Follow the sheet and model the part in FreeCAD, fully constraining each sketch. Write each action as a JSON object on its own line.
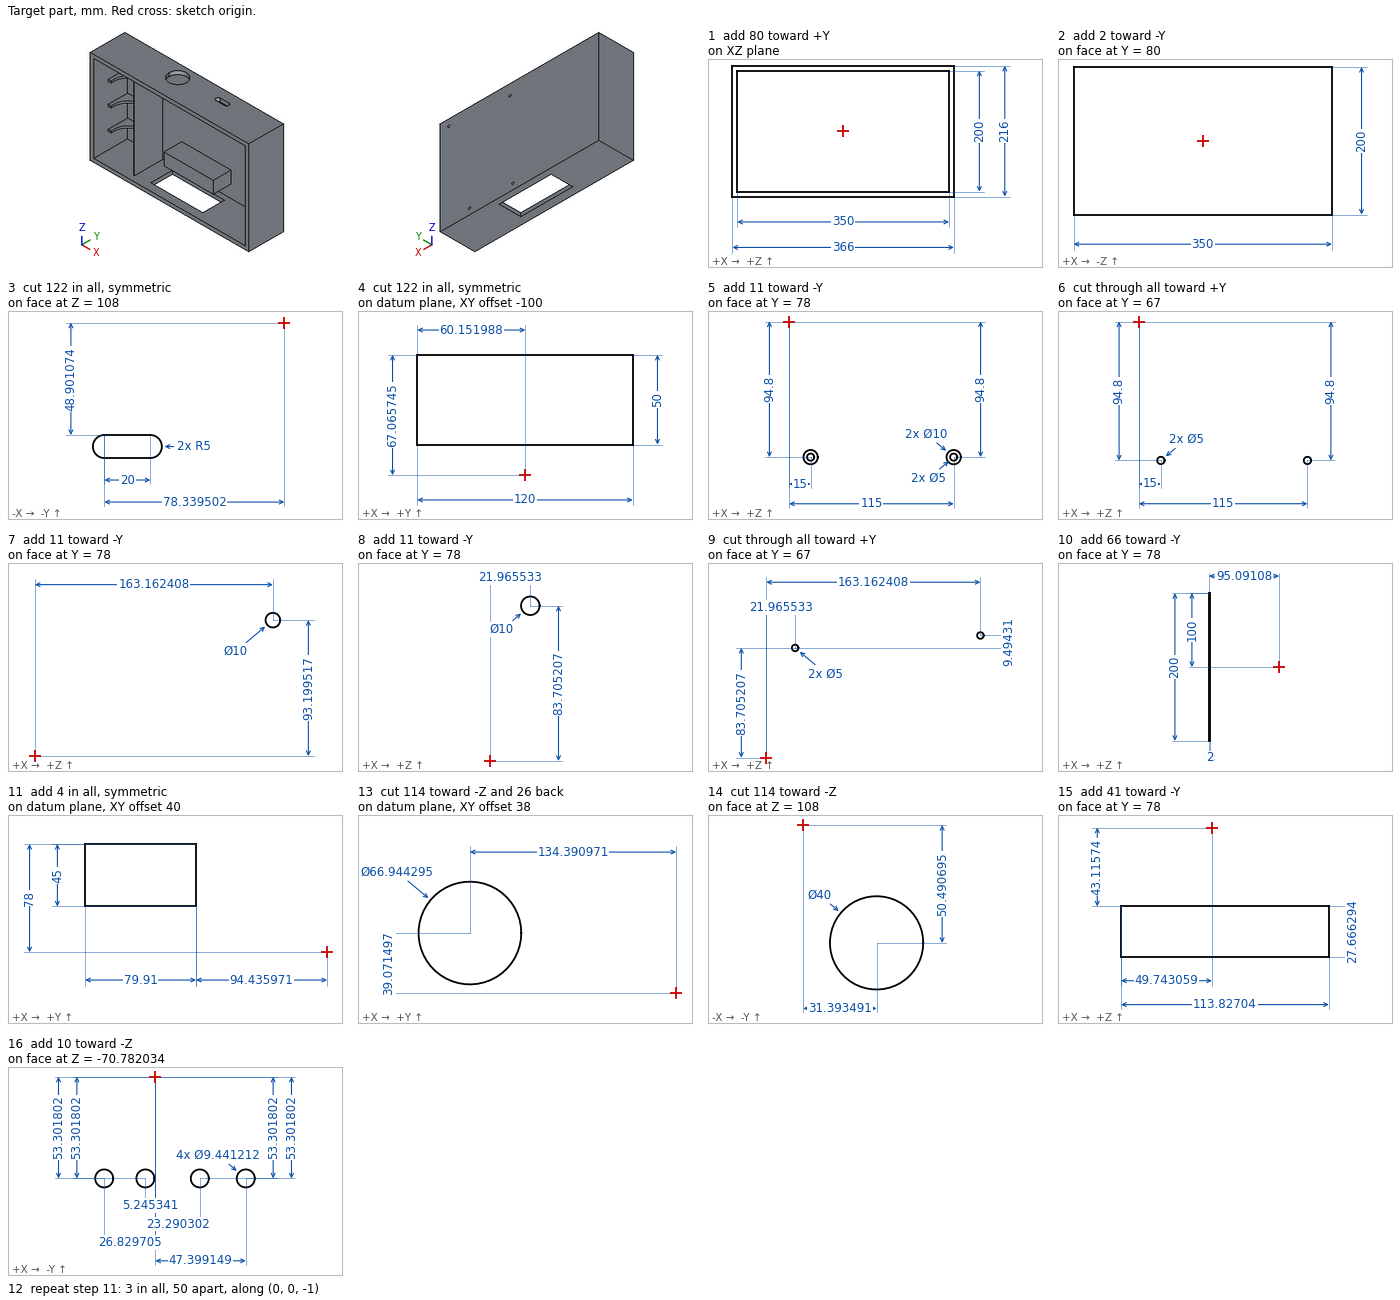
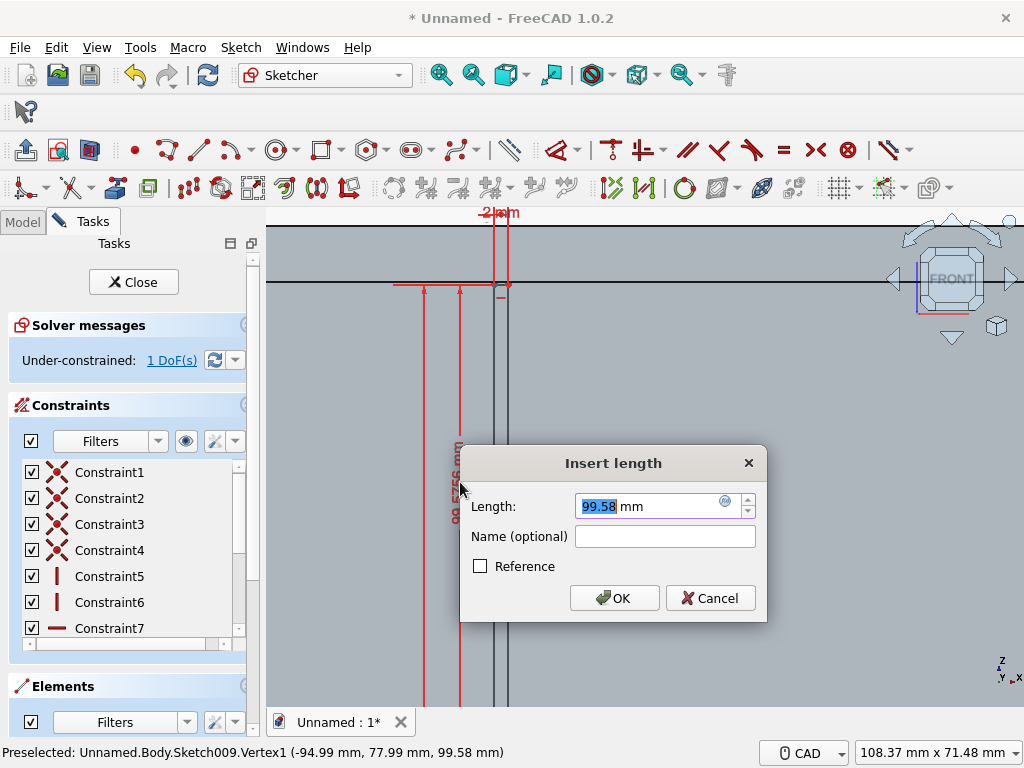
{"action": "type", "text": "100"}
{"action": "key", "text": "Return"}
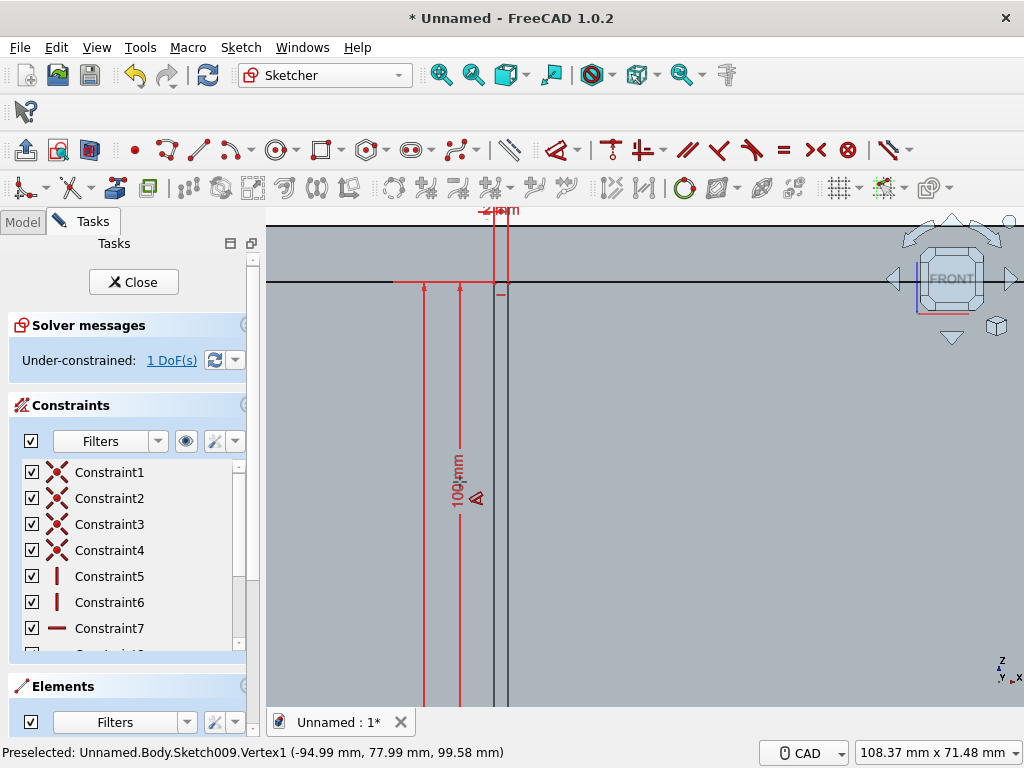
{"action": "left_click", "coordinate": [494, 282]}
{"action": "left_click", "coordinate": [677, 248]}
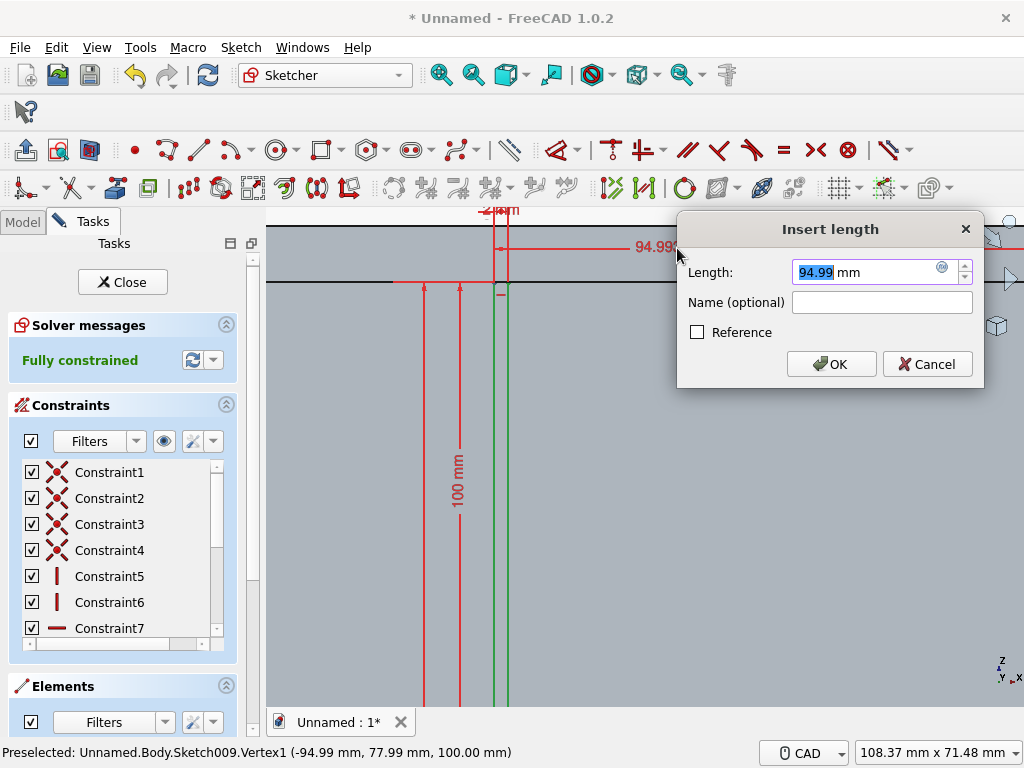
{"action": "type", "text": "95.09108"}
{"action": "key", "text": "Return"}
{"action": "key", "text": "Escape"}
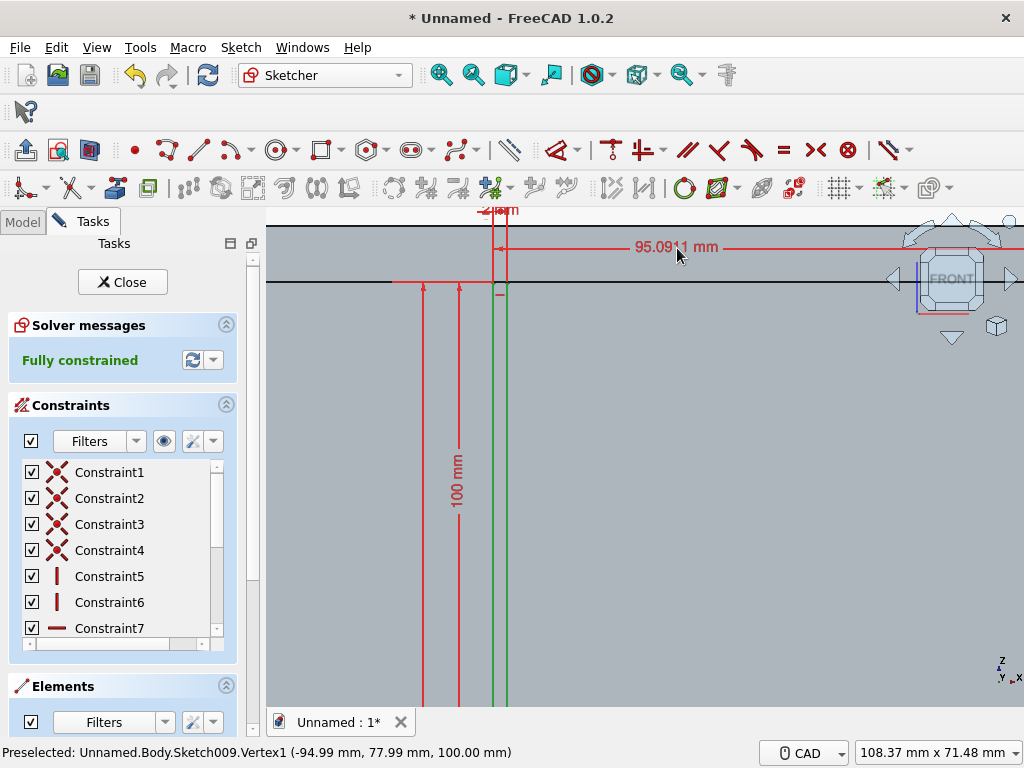
{"action": "left_click", "coordinate": [123, 282]}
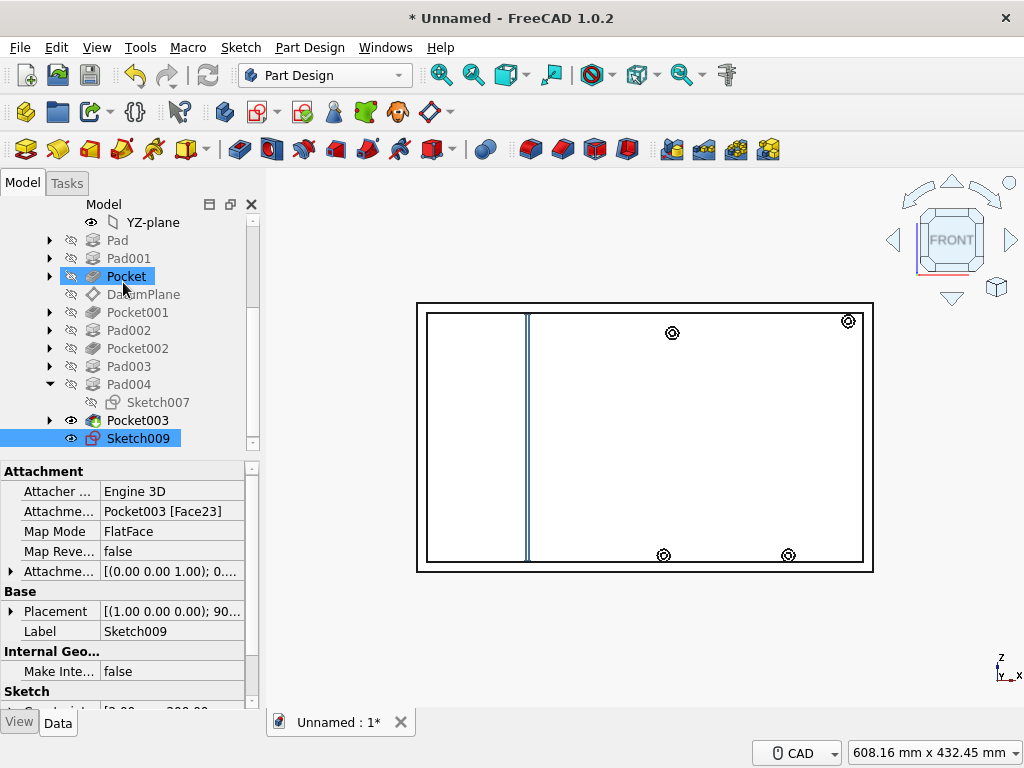
{"action": "left_click", "coordinate": [26, 150]}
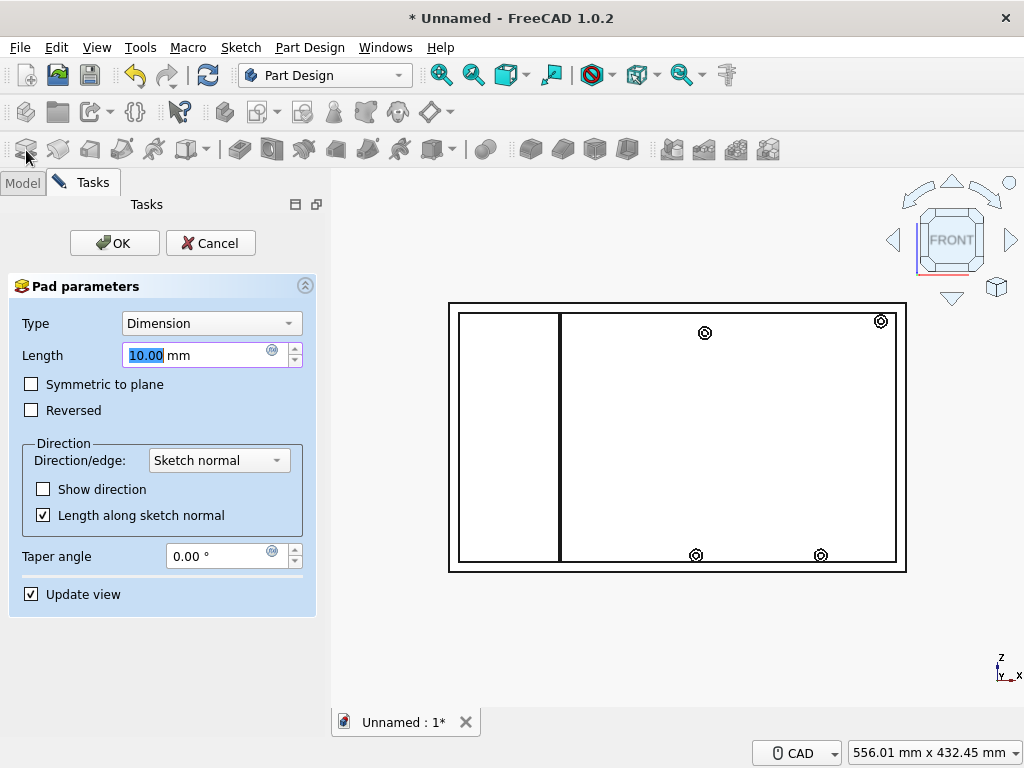
{"action": "type", "text": "66"}
{"action": "key", "text": "Tab"}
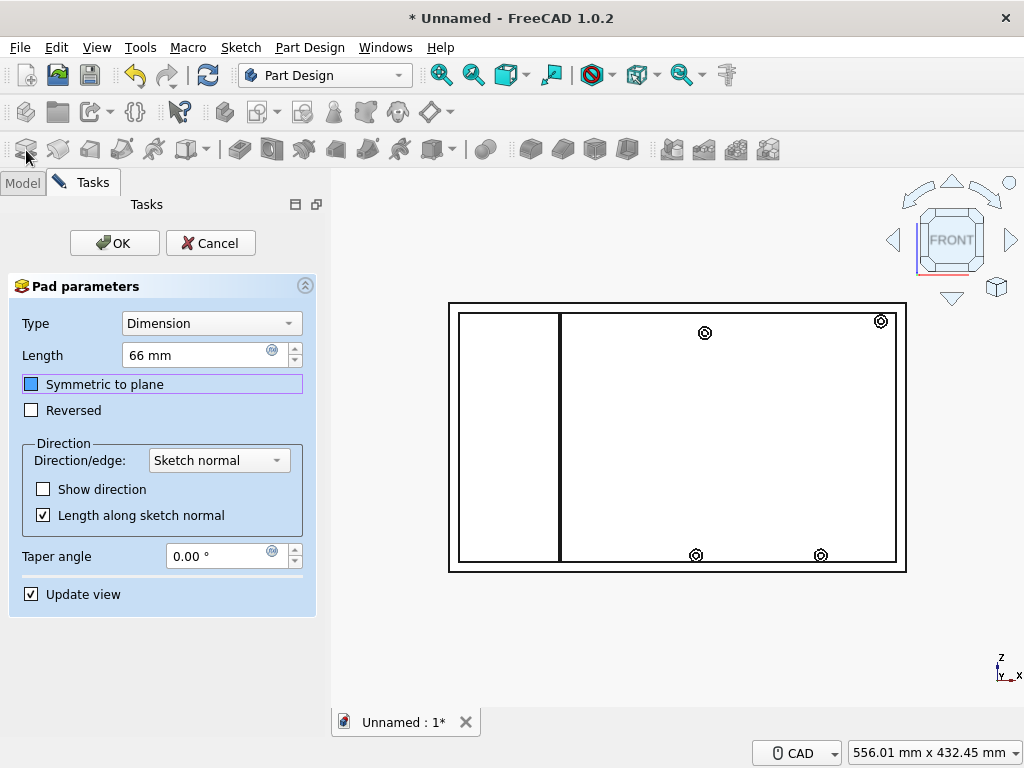
{"action": "left_click", "coordinate": [115, 243]}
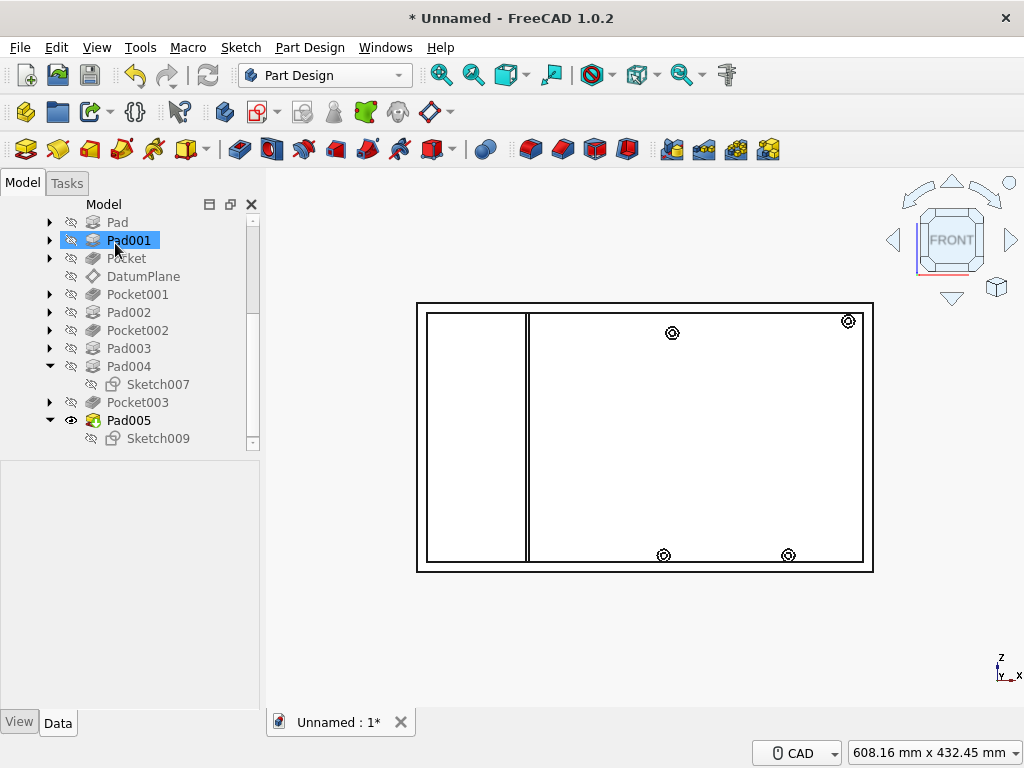
{"action": "scroll", "coordinate": [140, 326], "scroll_direction": "down", "scroll_amount": 3}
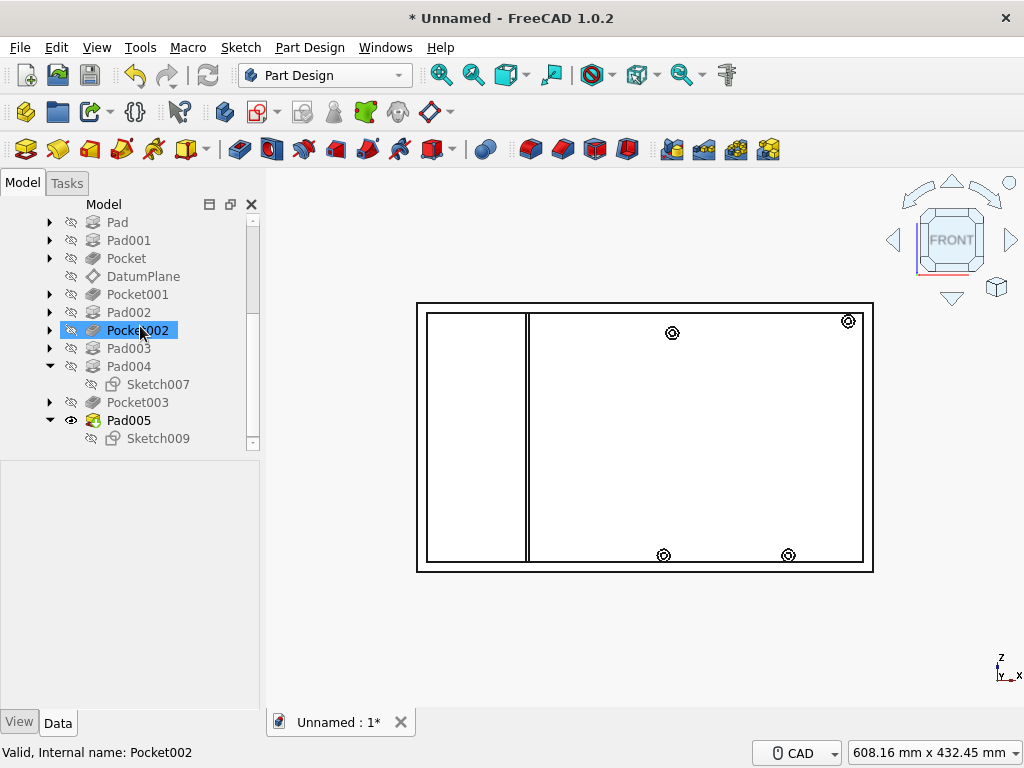
{"action": "scroll", "coordinate": [140, 326], "scroll_direction": "up", "scroll_amount": 15}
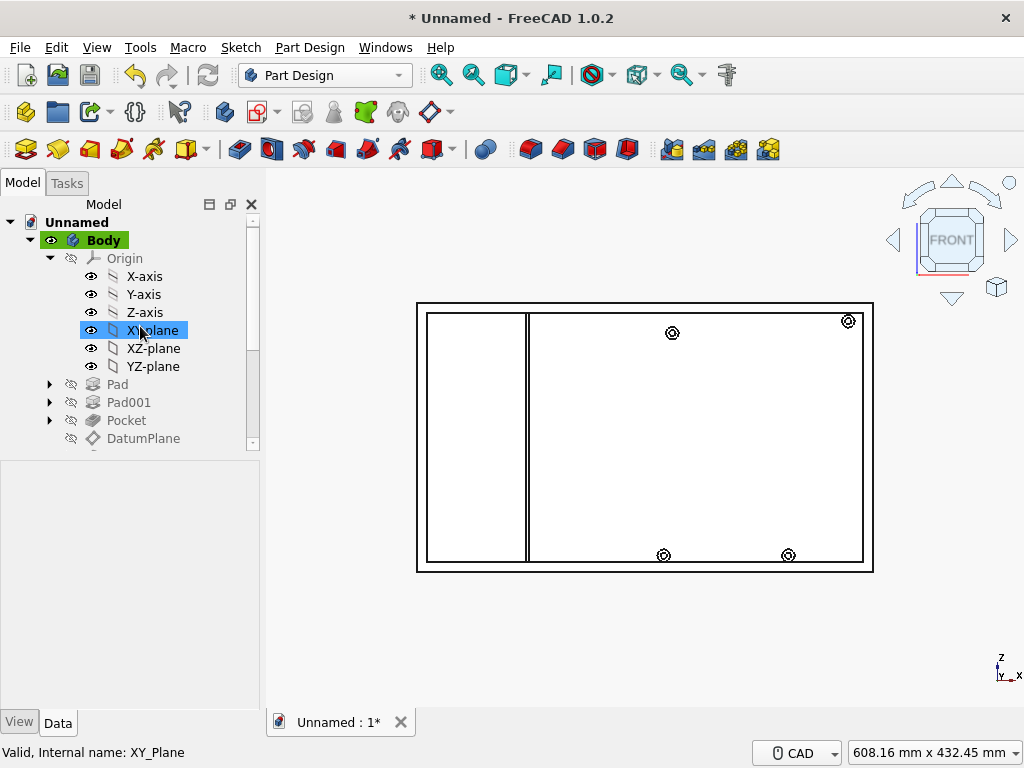
{"action": "left_click", "coordinate": [136, 330]}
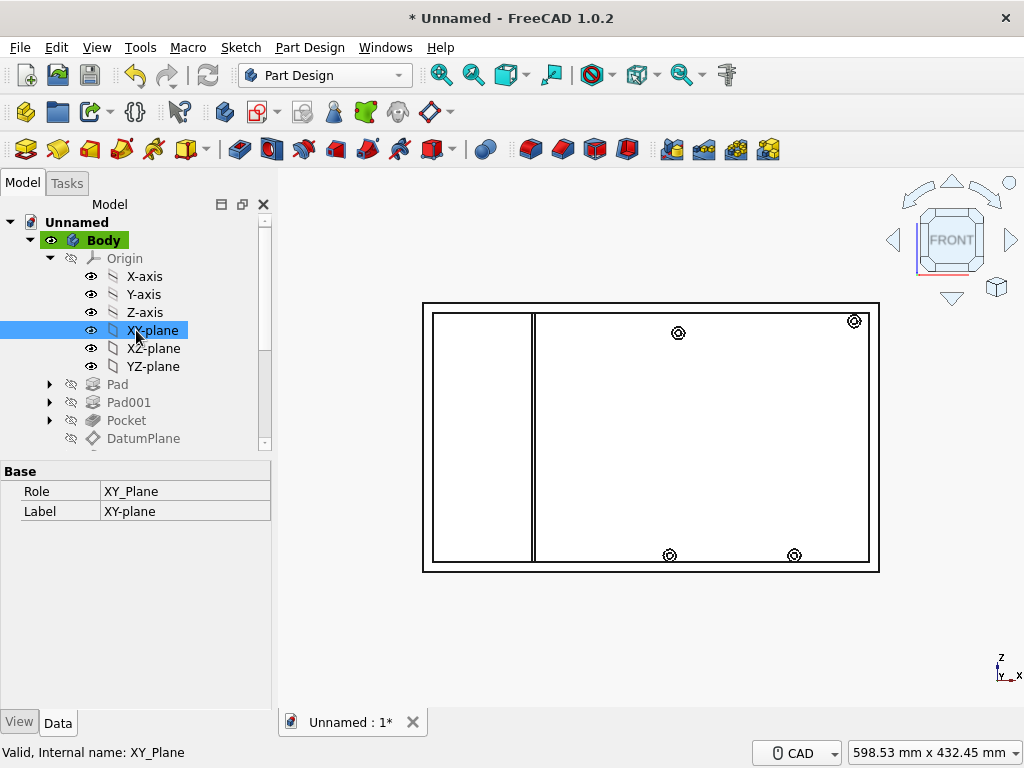
{"action": "left_click", "coordinate": [430, 112]}